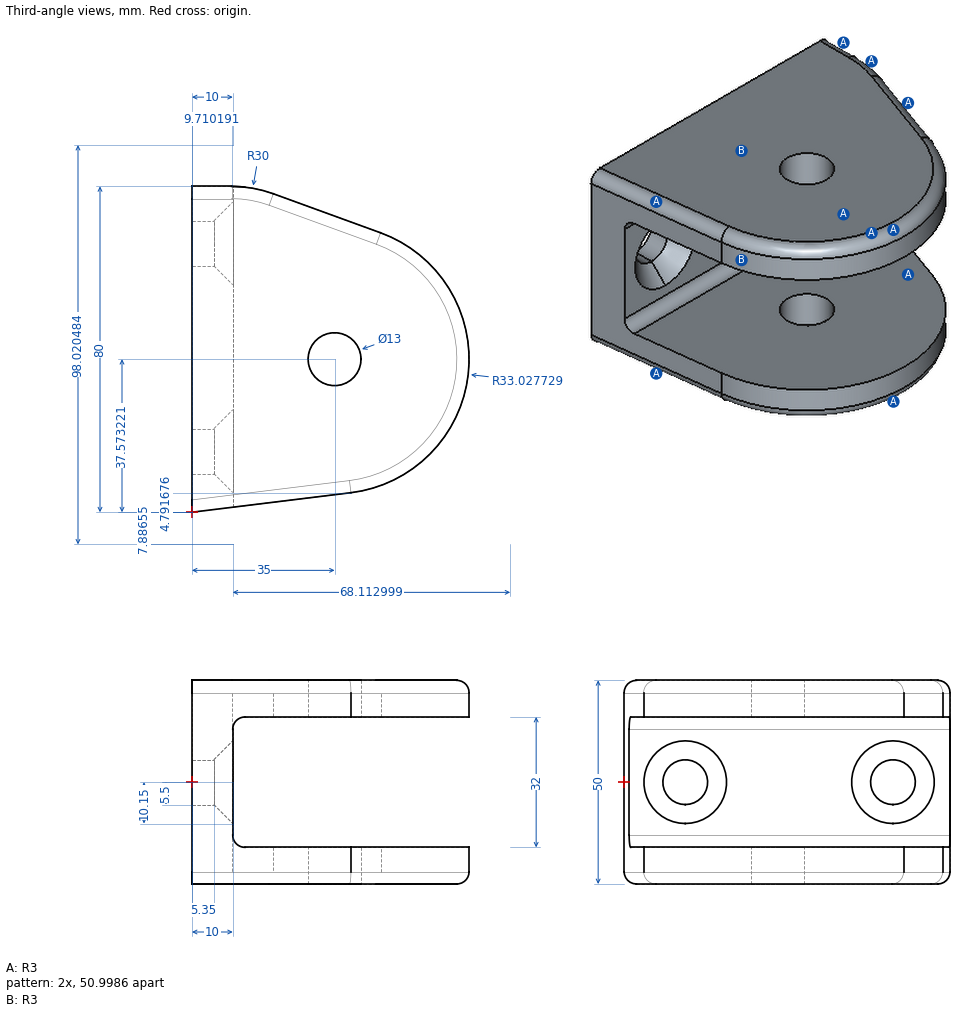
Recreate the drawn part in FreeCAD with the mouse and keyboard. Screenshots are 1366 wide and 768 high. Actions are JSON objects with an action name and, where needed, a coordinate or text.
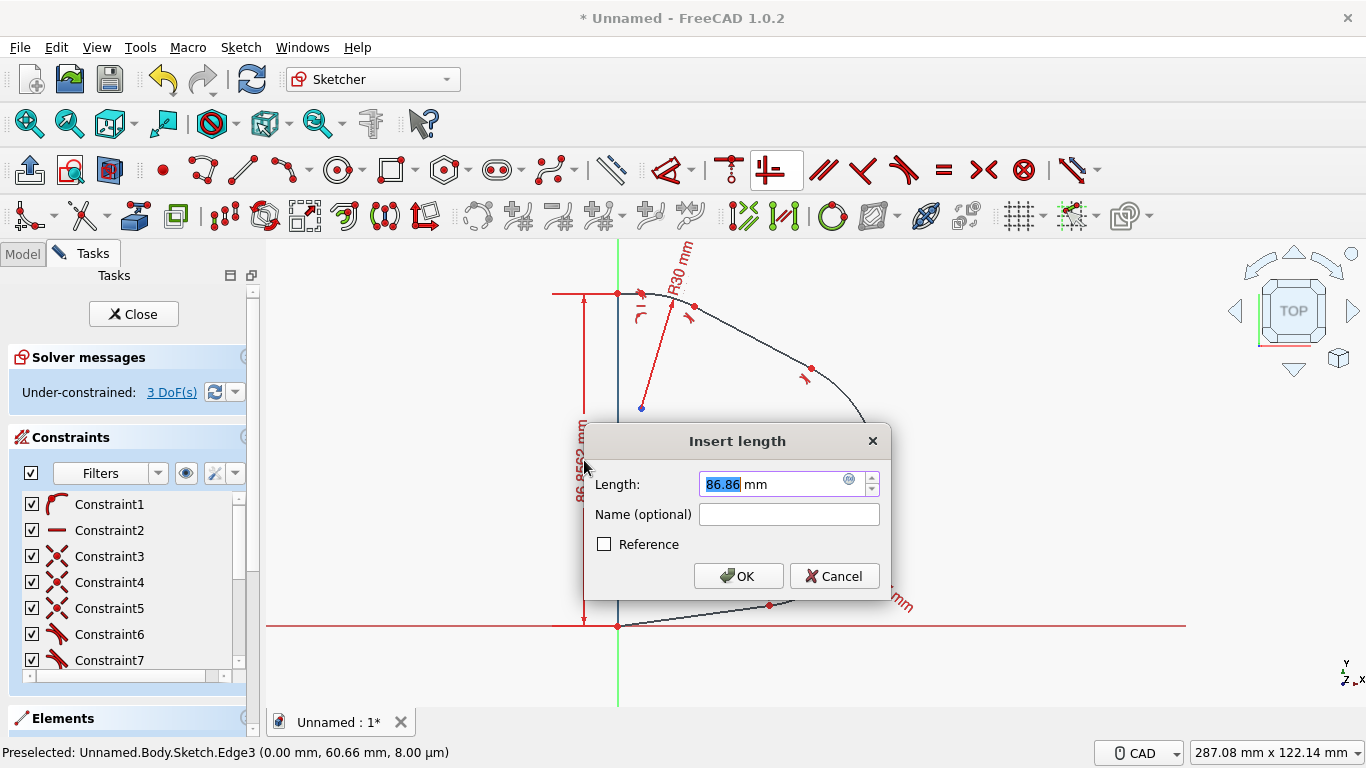
{"action": "type", "text": "80"}
{"action": "key", "text": "Return"}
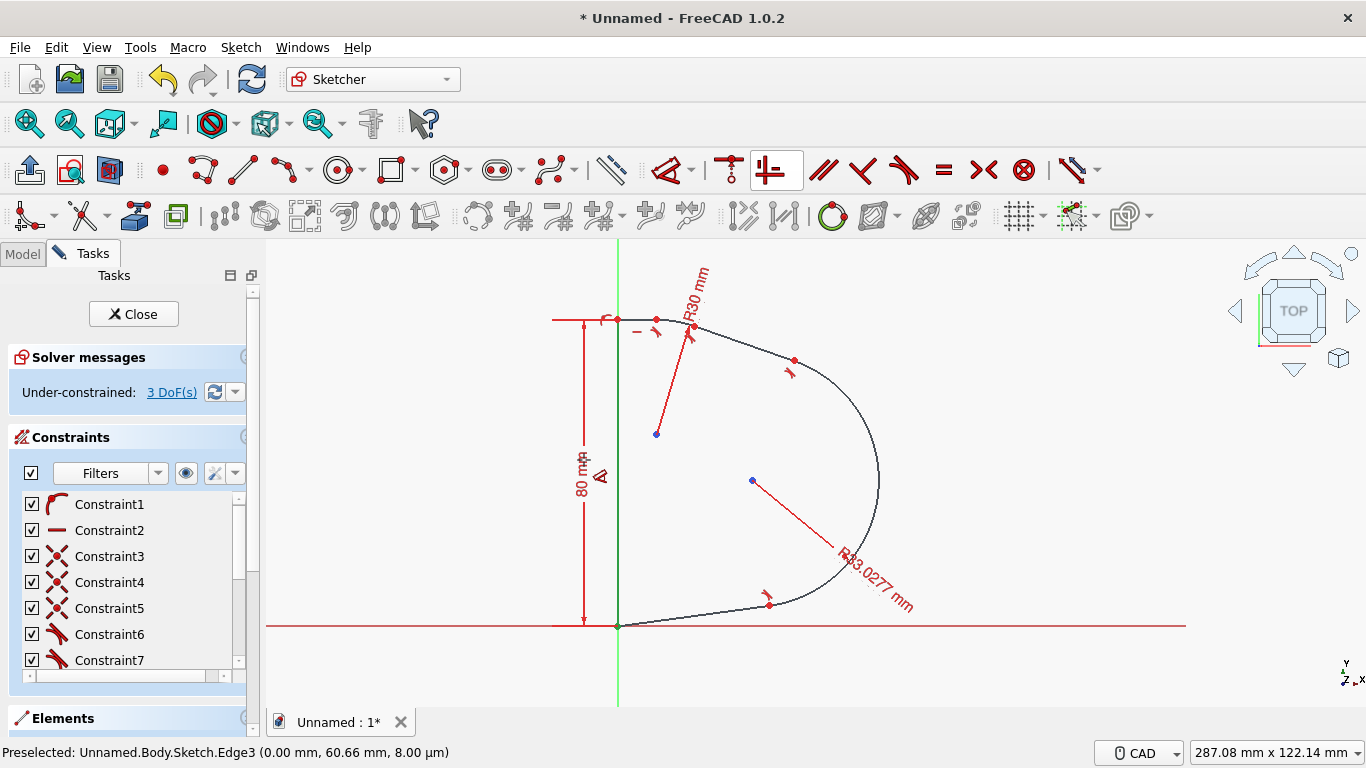
{"action": "left_click", "coordinate": [752, 480]}
{"action": "left_click", "coordinate": [685, 660]}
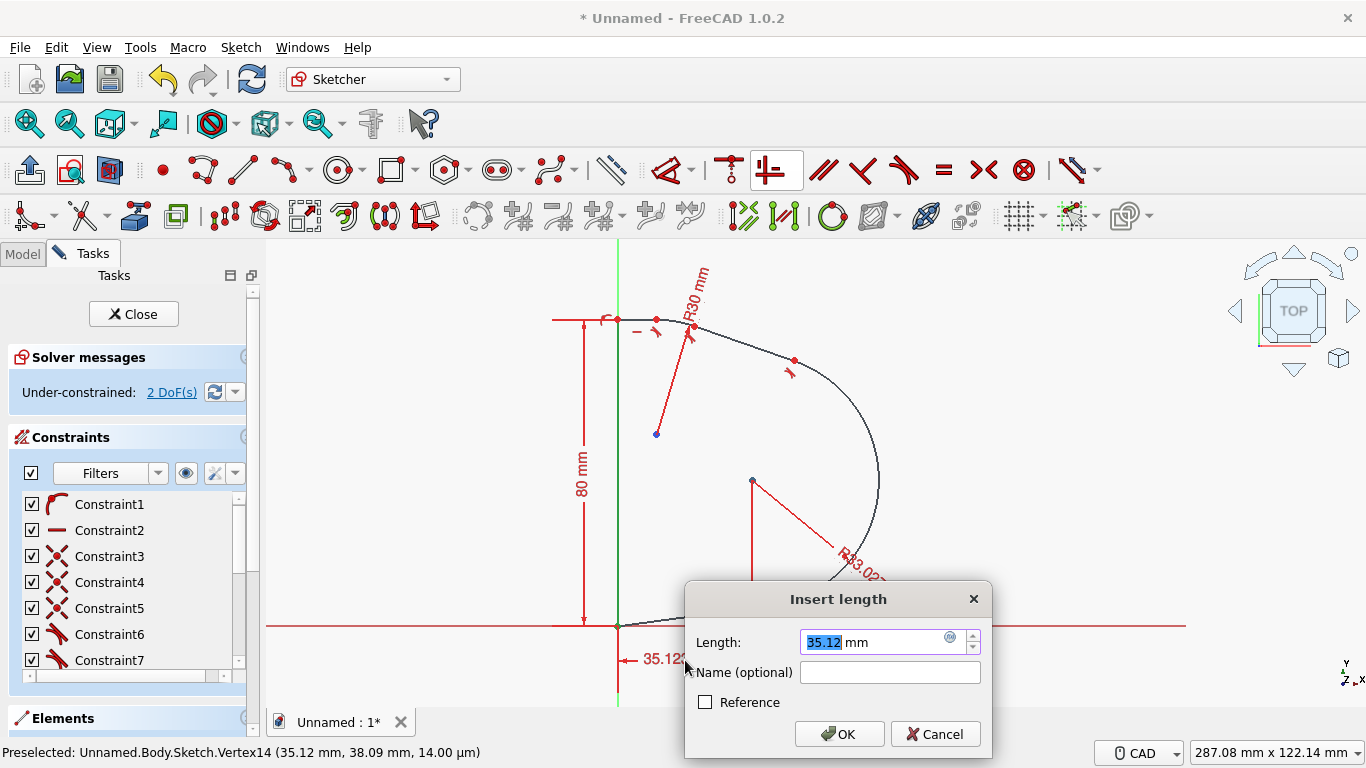
{"action": "type", "text": "35"}
{"action": "key", "text": "Return"}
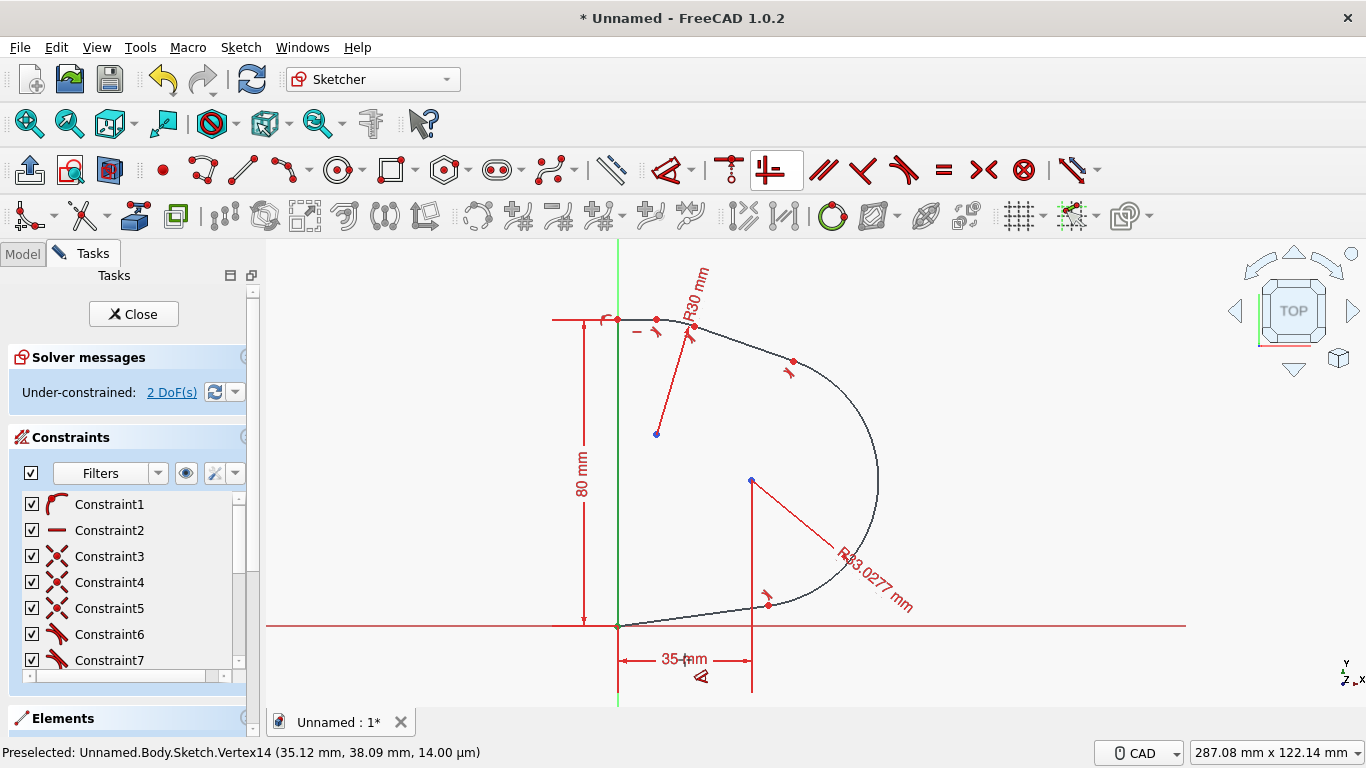
{"action": "left_click", "coordinate": [645, 320]}
{"action": "left_click", "coordinate": [637, 354]}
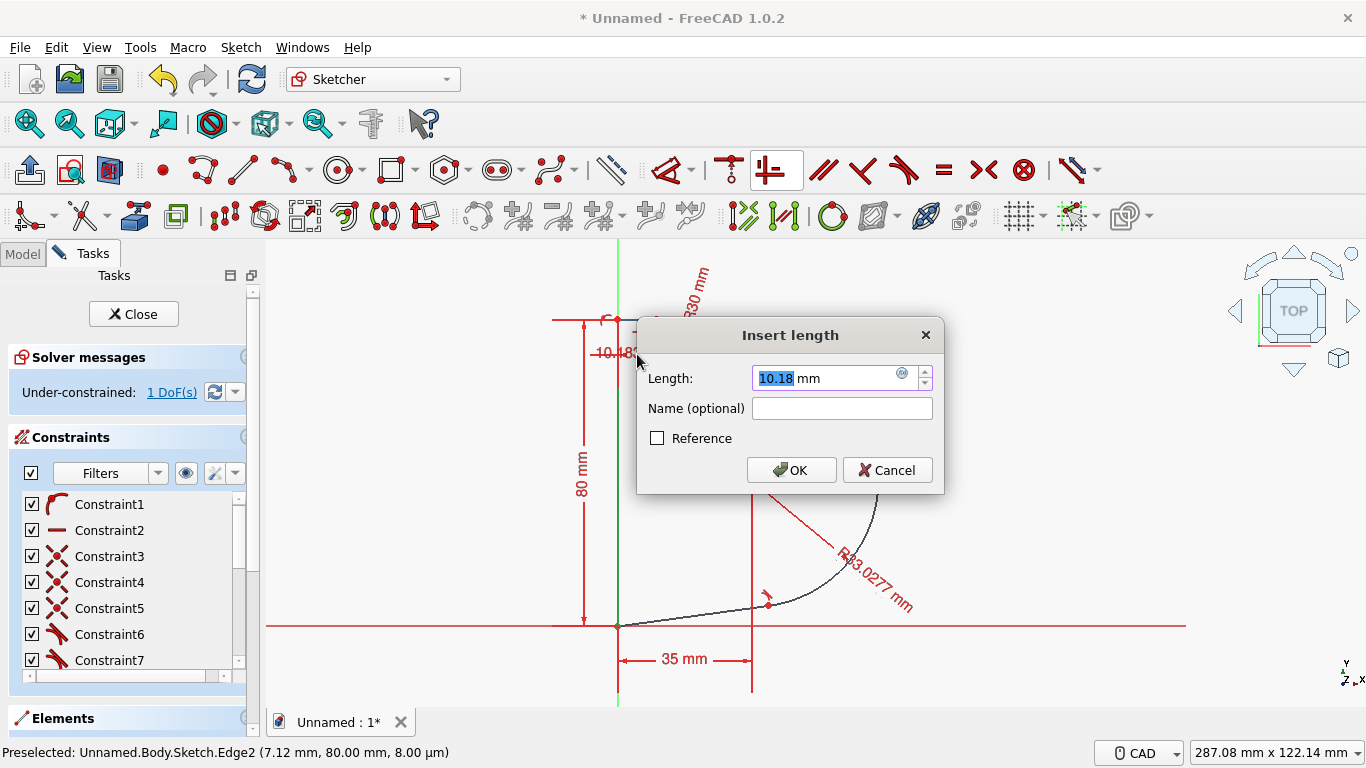
{"action": "type", "text": "9.710191"}
{"action": "key", "text": "Return"}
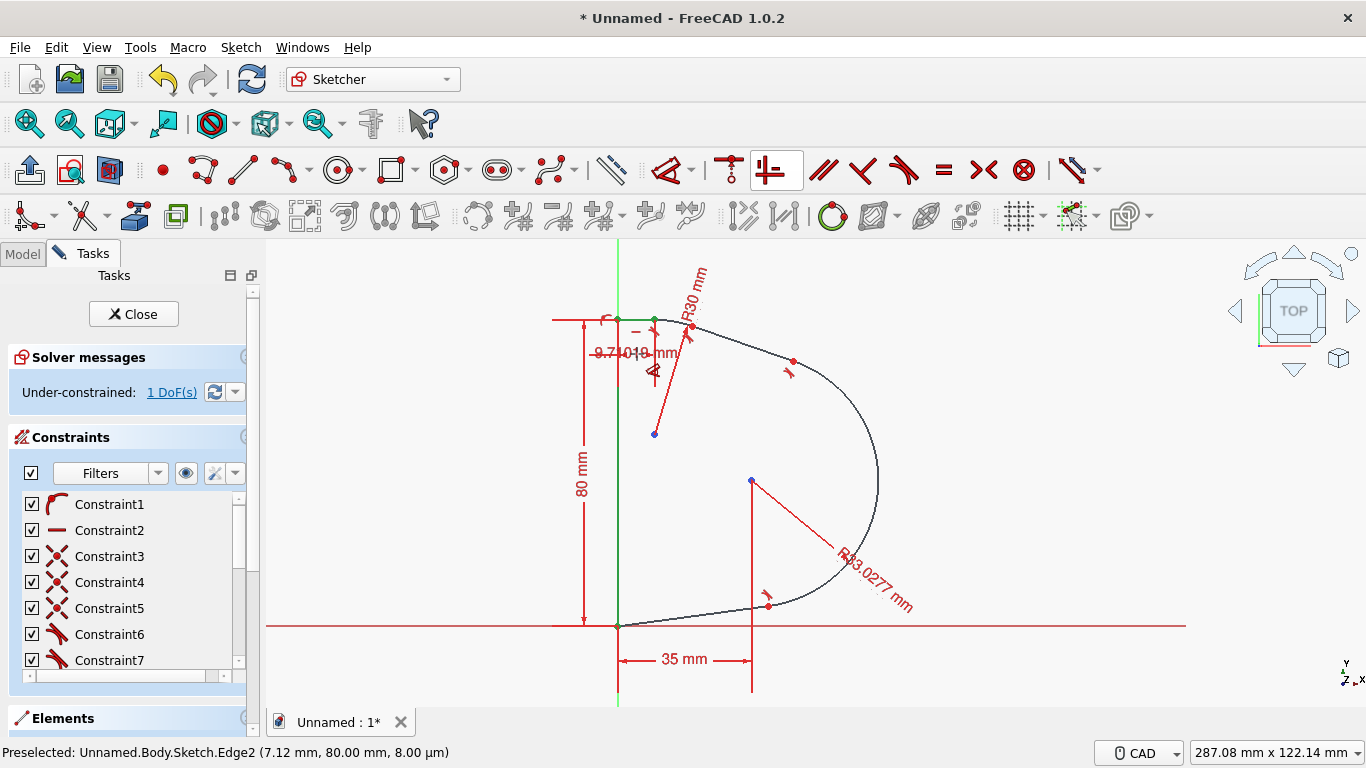
{"action": "scroll", "coordinate": [769, 606], "scroll_direction": "up", "scroll_amount": 4}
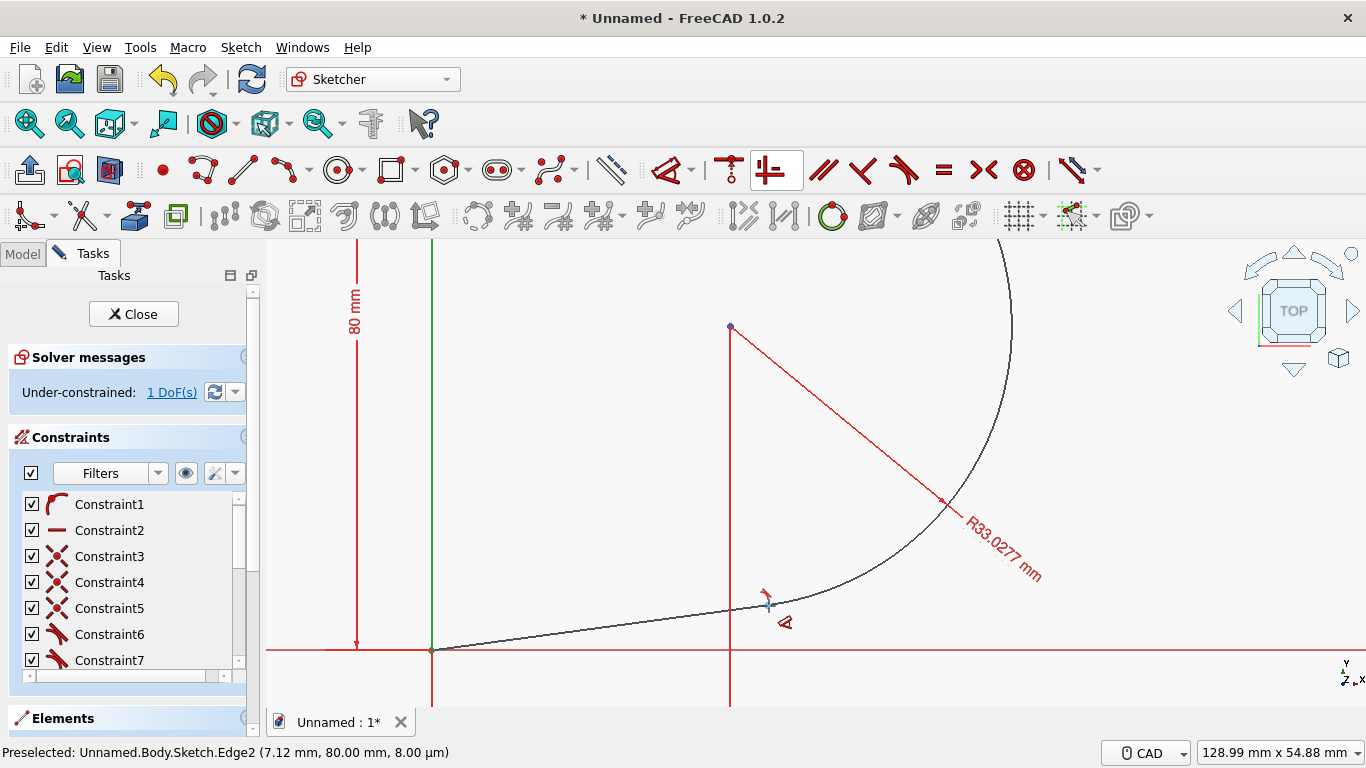
{"action": "left_click", "coordinate": [768, 605]}
{"action": "left_click", "coordinate": [398, 628]}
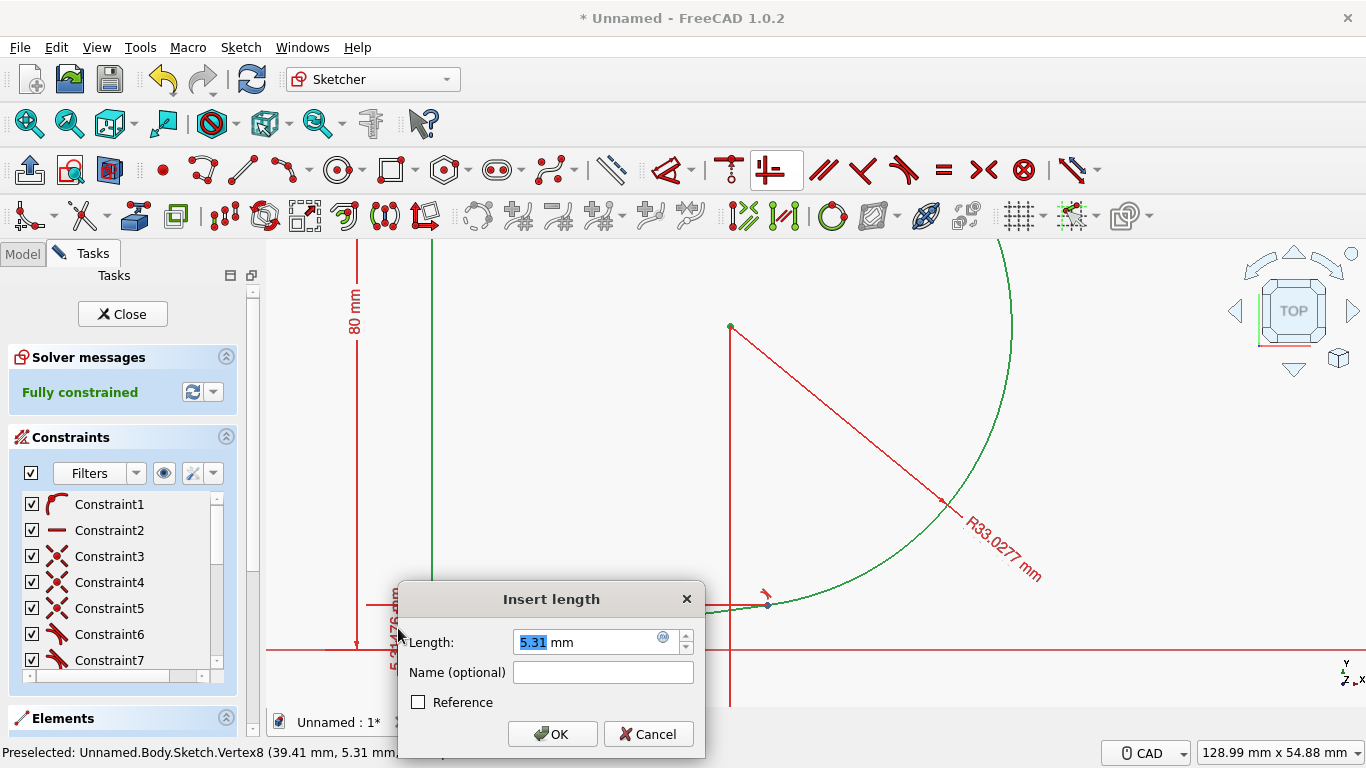
{"action": "type", "text": "4.791676"}
{"action": "key", "text": "Return"}
{"action": "key", "text": "Escape"}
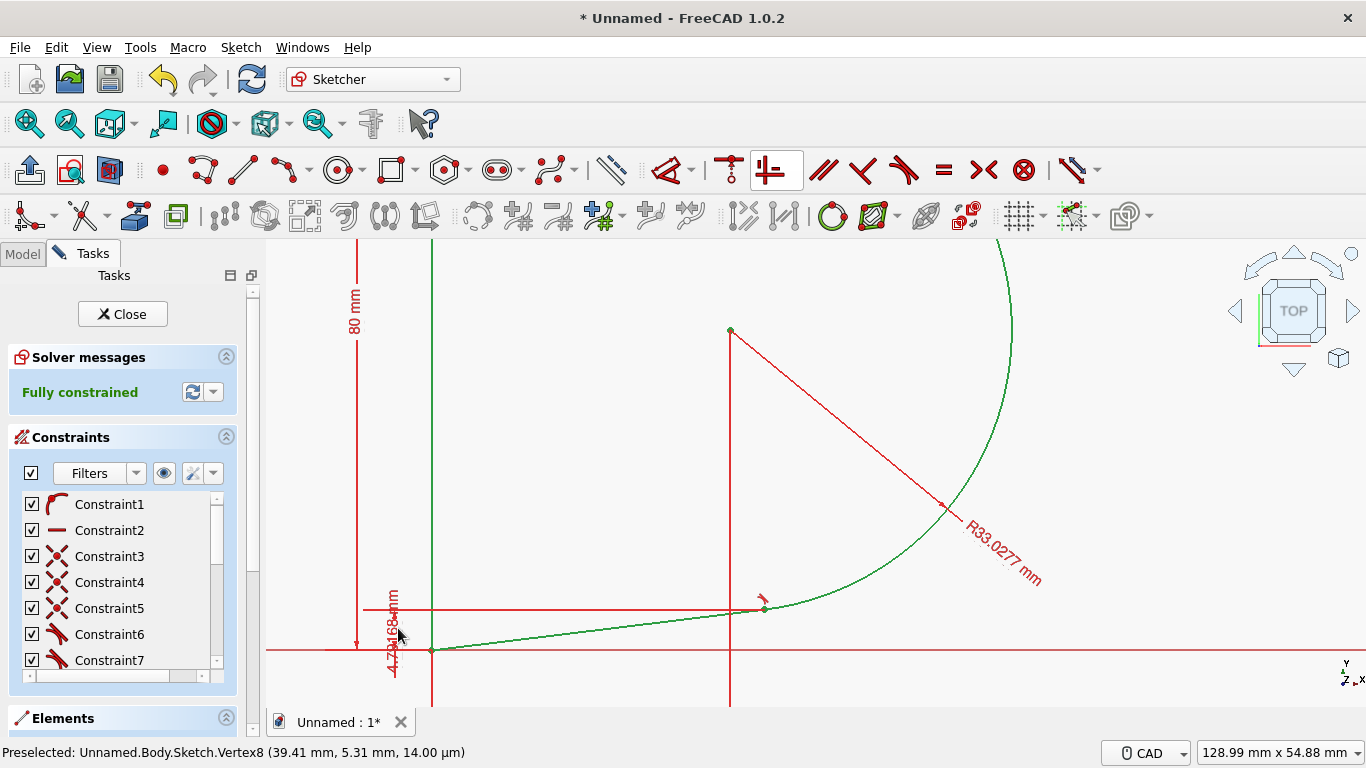
{"action": "left_click", "coordinate": [123, 314]}